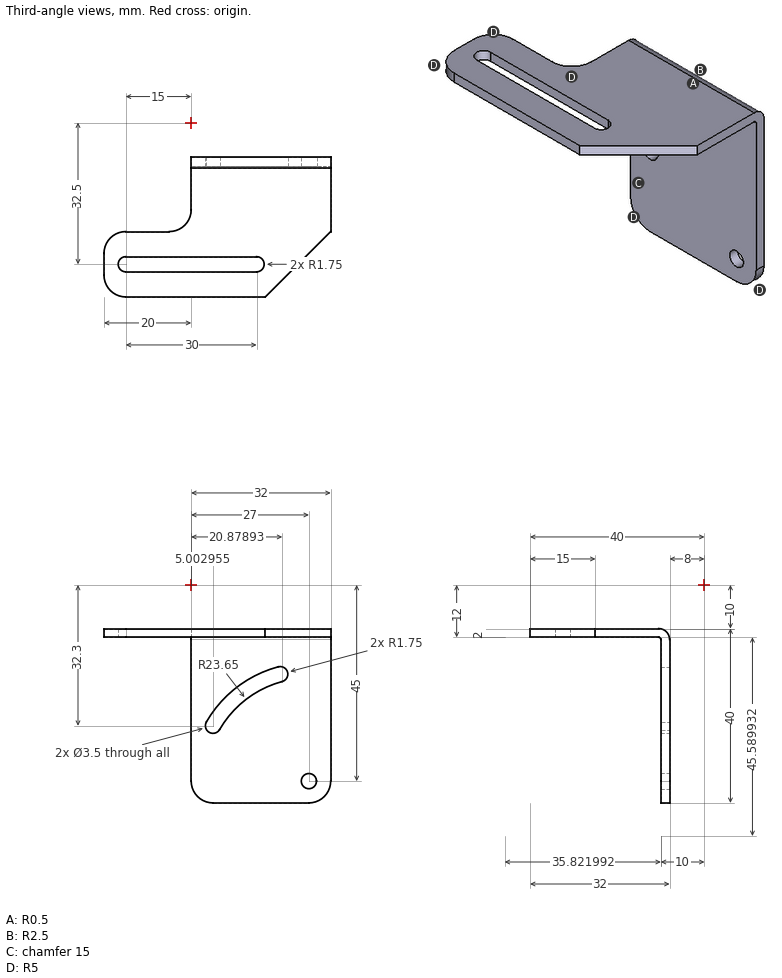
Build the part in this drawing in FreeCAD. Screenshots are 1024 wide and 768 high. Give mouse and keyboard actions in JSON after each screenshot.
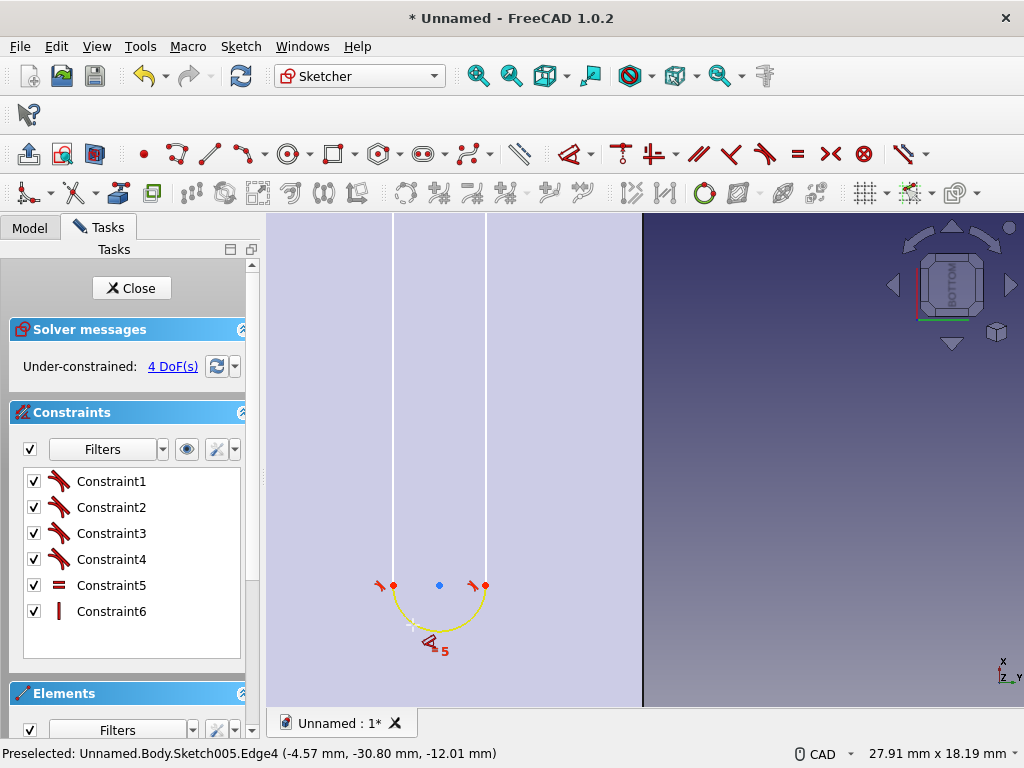
{"action": "left_click", "coordinate": [412, 623]}
{"action": "left_click", "coordinate": [393, 649]}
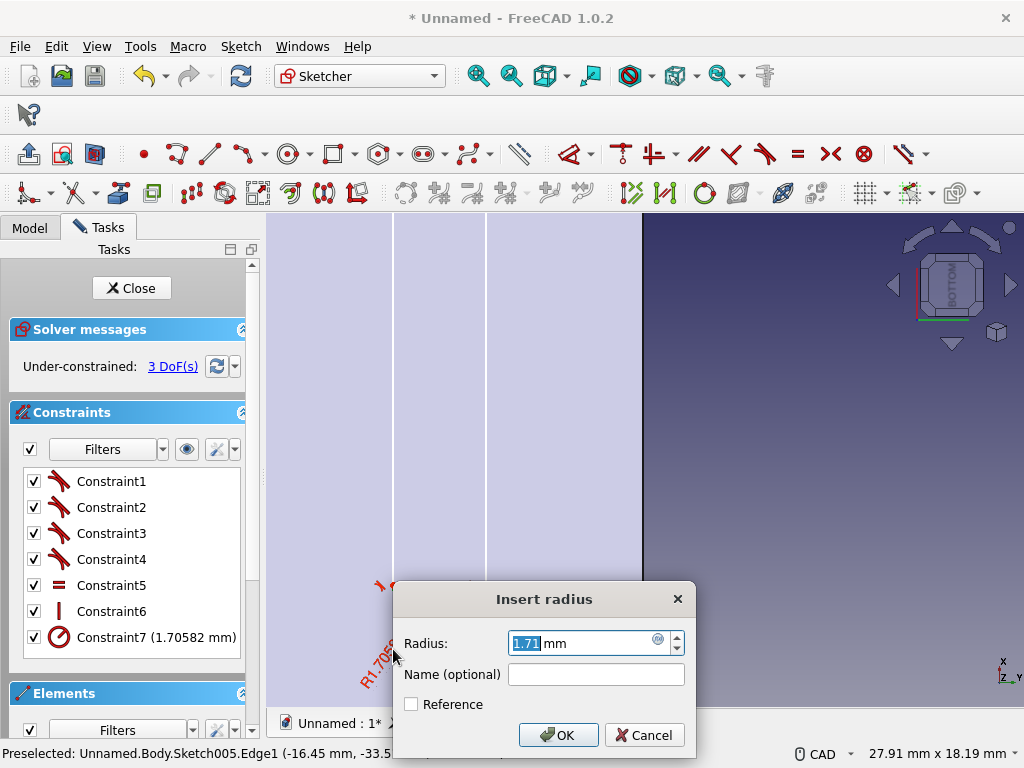
{"action": "type", "text": "1.75"}
{"action": "key", "text": "Return"}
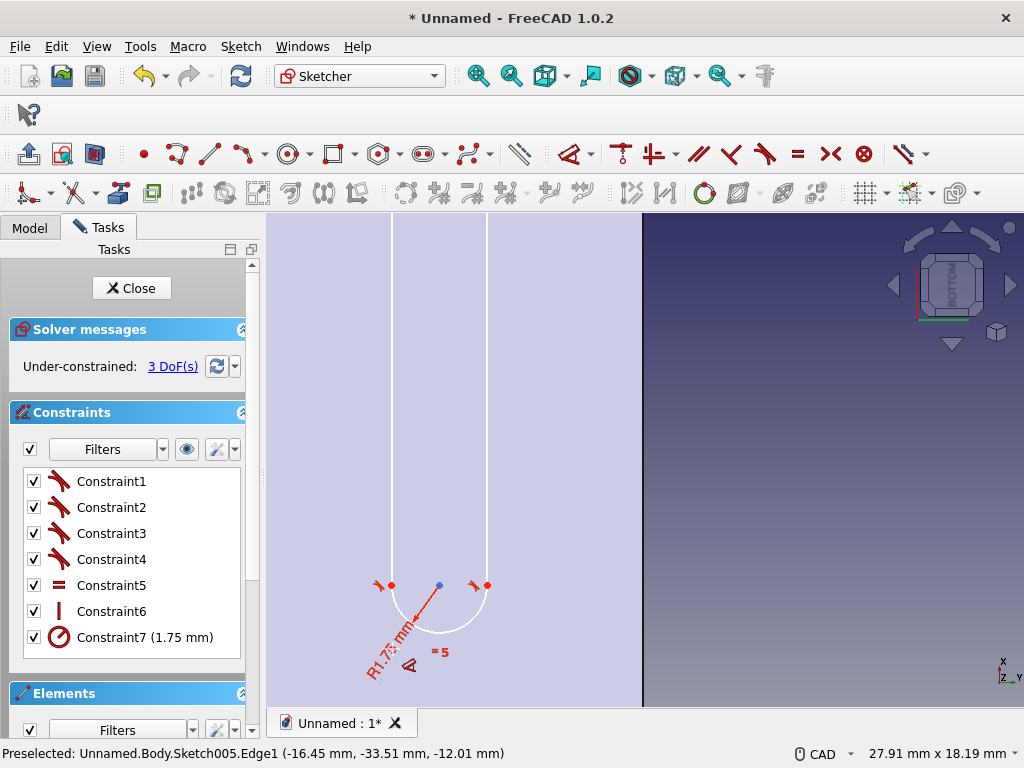
{"action": "left_click", "coordinate": [392, 341]}
{"action": "left_click", "coordinate": [358, 413]}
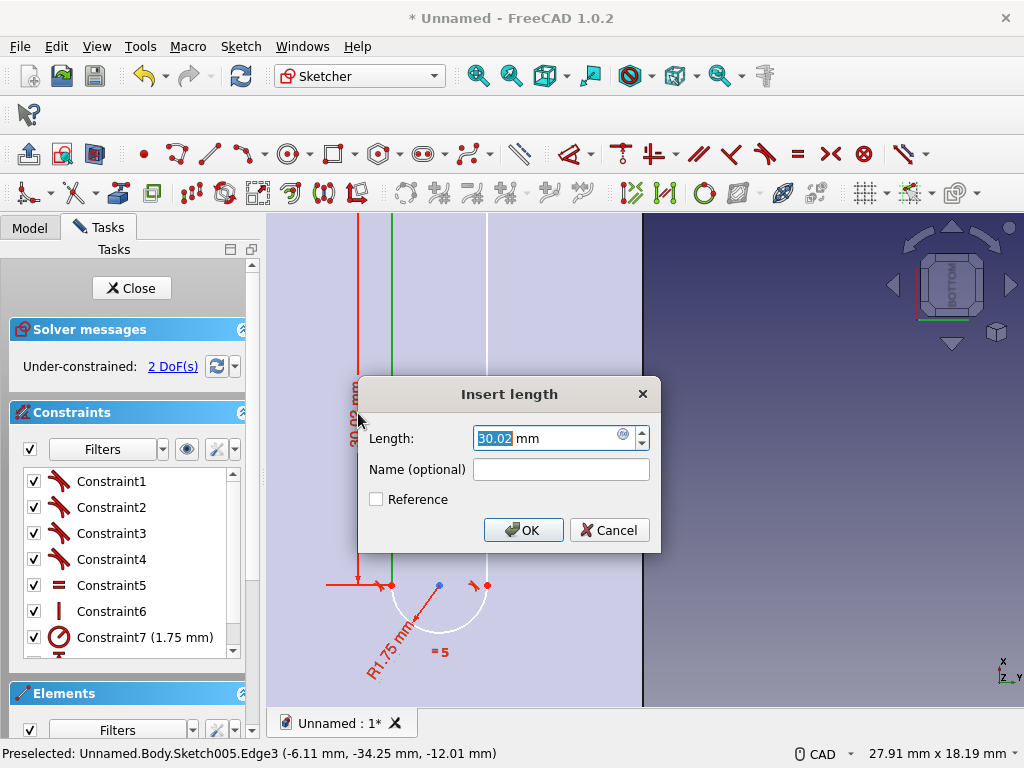
{"action": "type", "text": "30"}
{"action": "key", "text": "Return"}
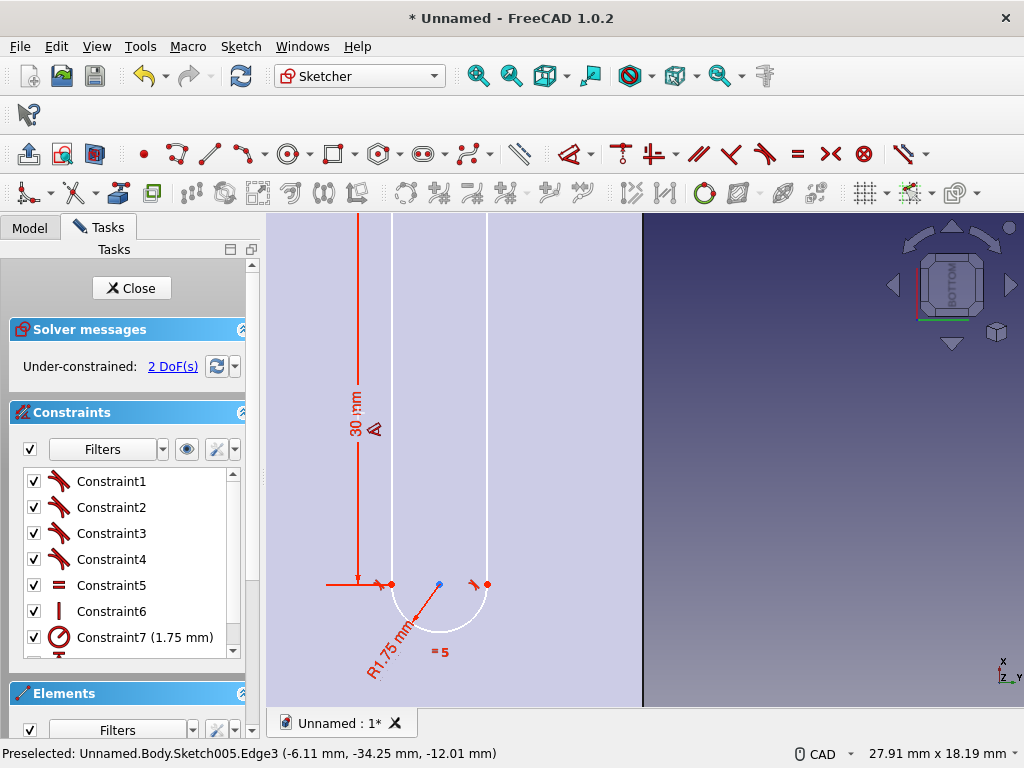
{"action": "left_click", "coordinate": [392, 585]}
{"action": "left_click", "coordinate": [358, 334]}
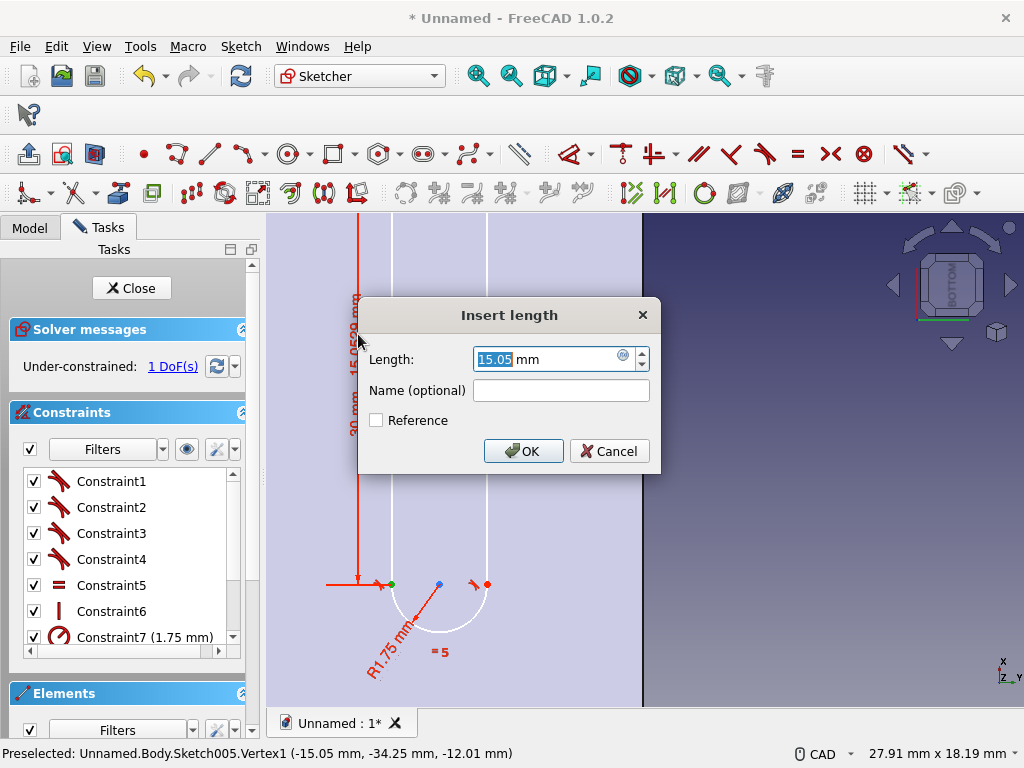
{"action": "type", "text": "15"}
{"action": "key", "text": "Return"}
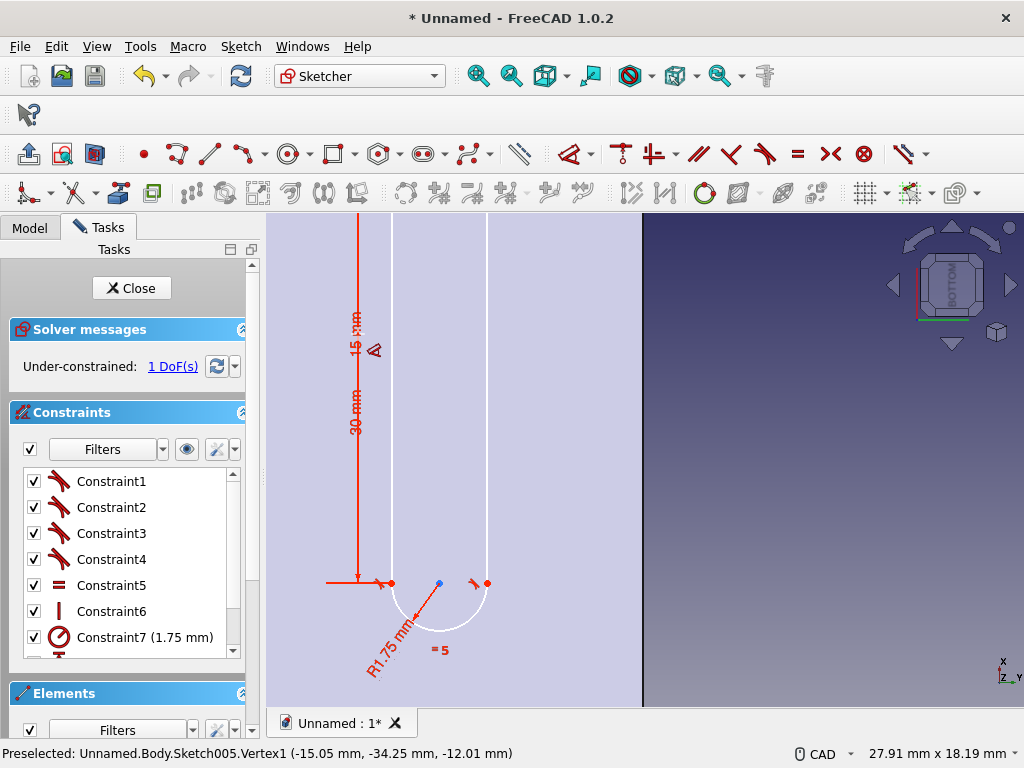
{"action": "left_click", "coordinate": [439, 583]}
{"action": "left_click", "coordinate": [649, 617]}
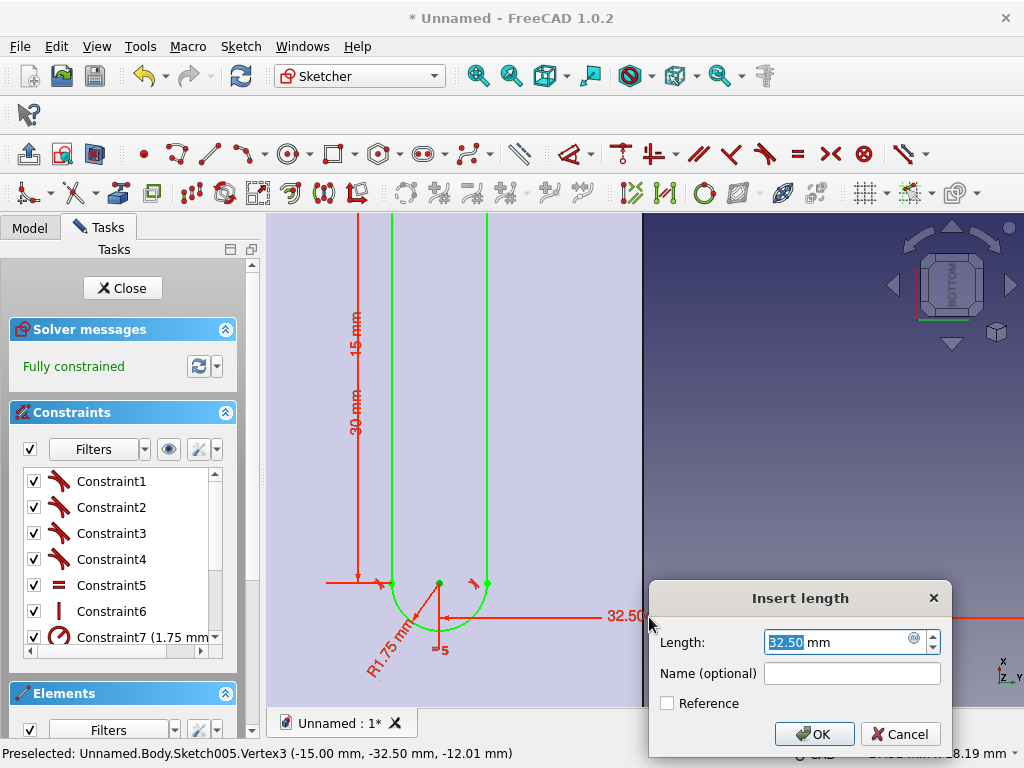
{"action": "type", "text": "32.5"}
{"action": "key", "text": "Return"}
{"action": "key", "text": "Escape"}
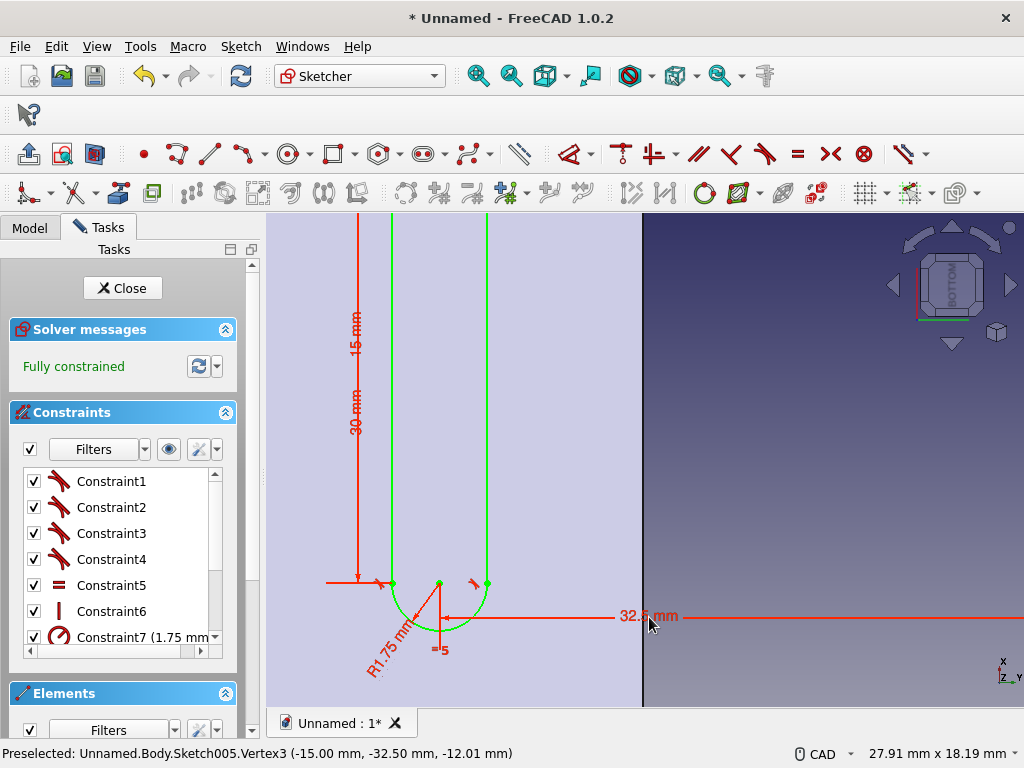
{"action": "left_click", "coordinate": [123, 288]}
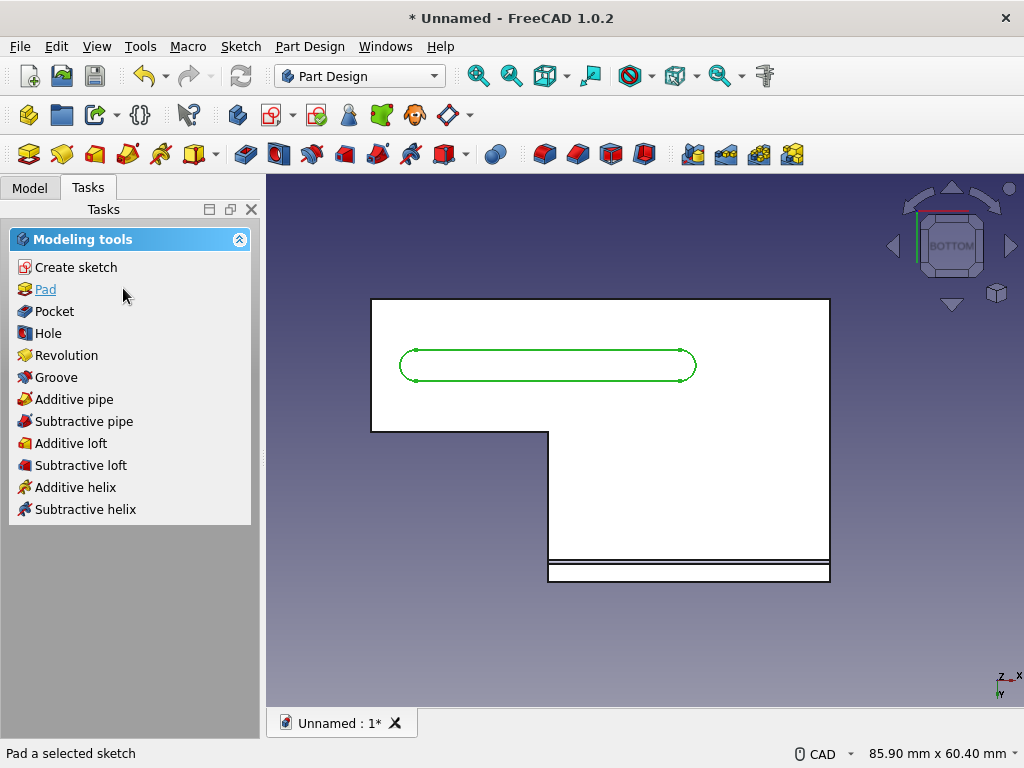
{"action": "left_click", "coordinate": [246, 154]}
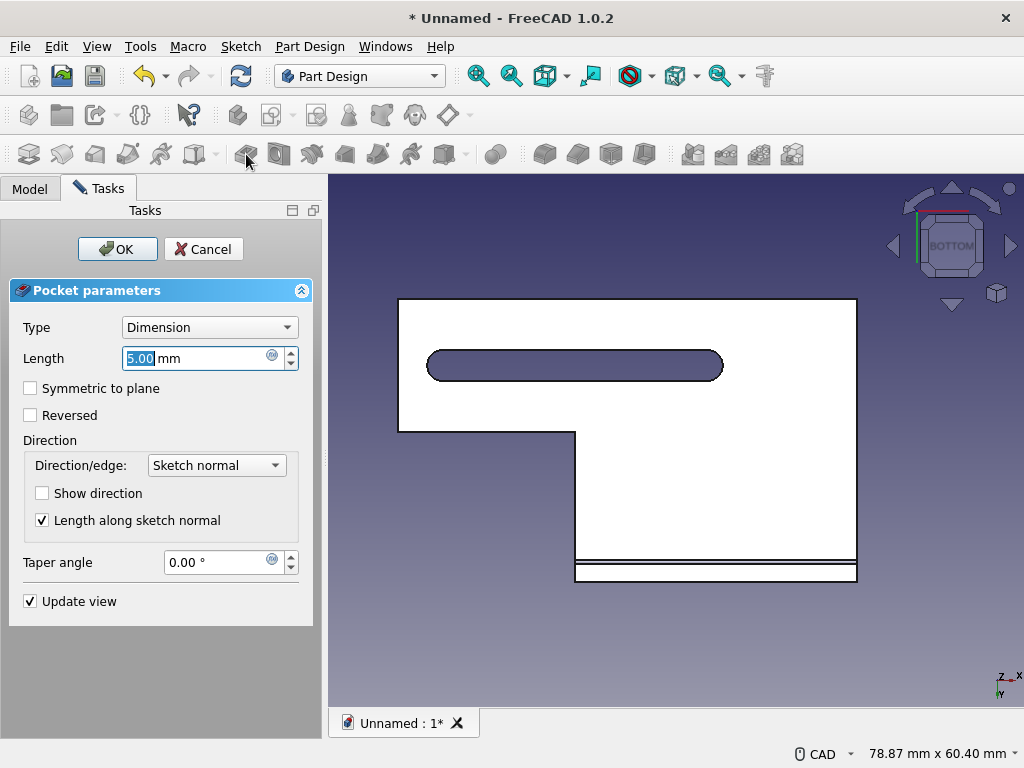
{"action": "left_click", "coordinate": [210, 328]}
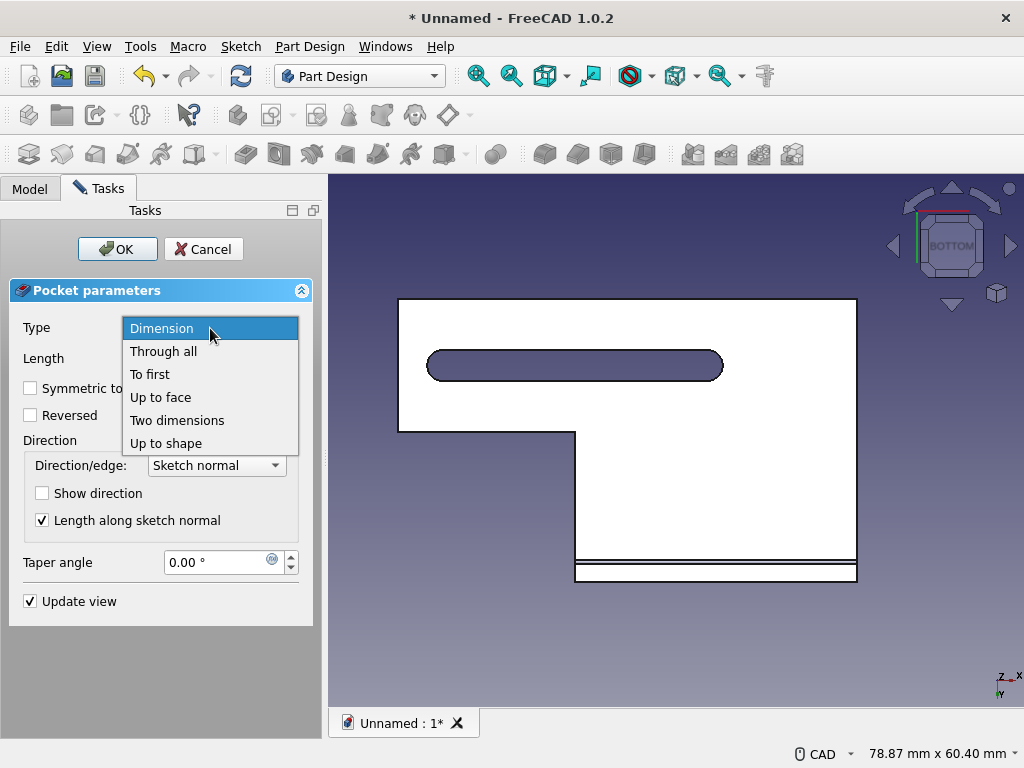
{"action": "left_click", "coordinate": [208, 352]}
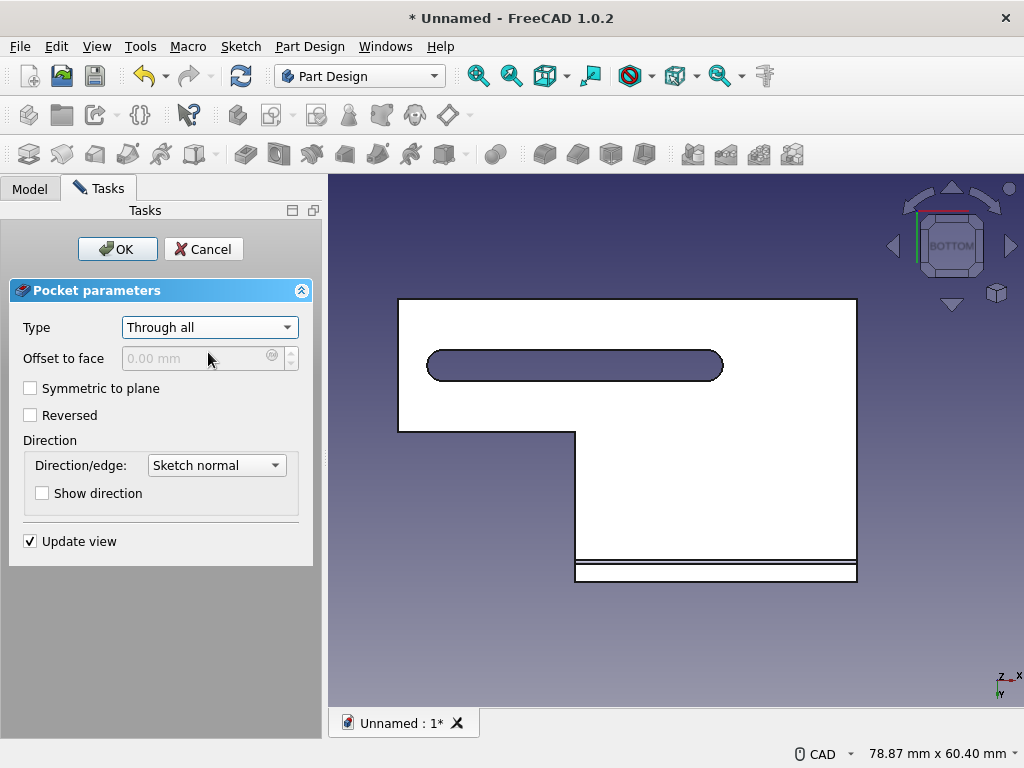
{"action": "left_click", "coordinate": [118, 249]}